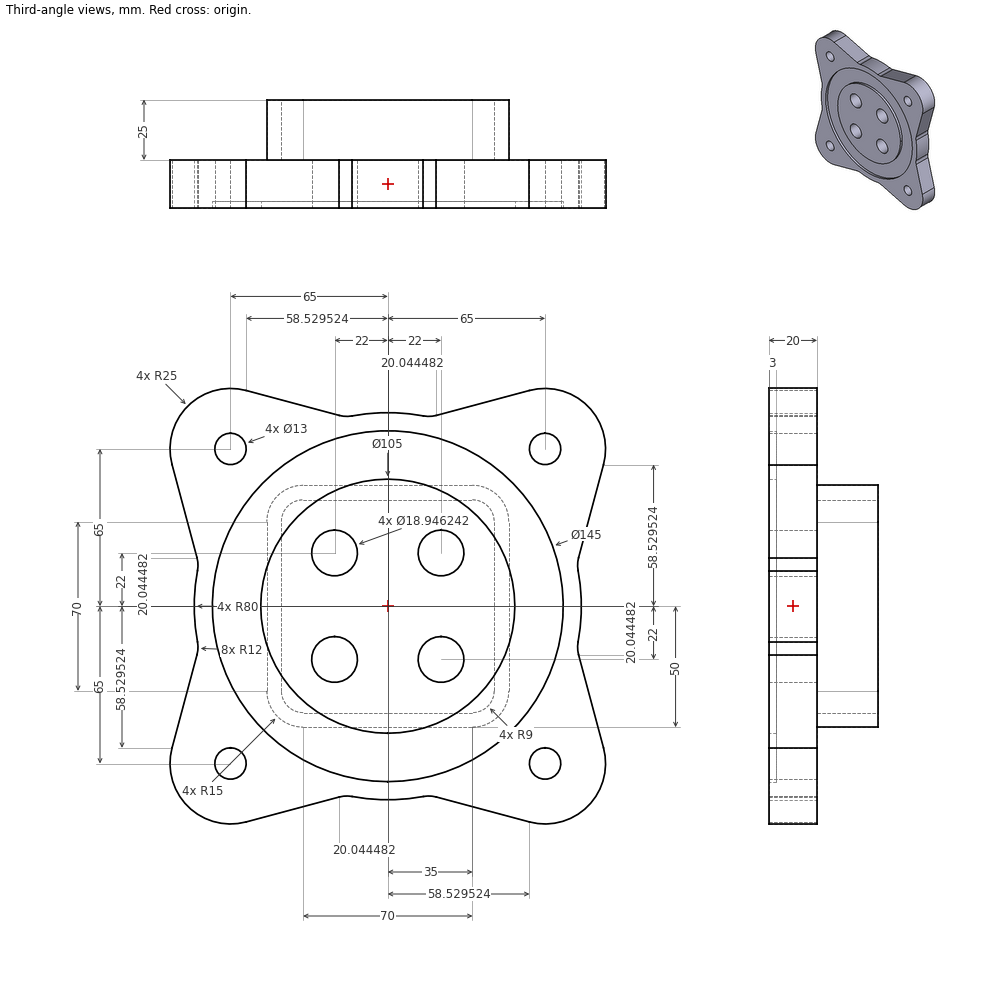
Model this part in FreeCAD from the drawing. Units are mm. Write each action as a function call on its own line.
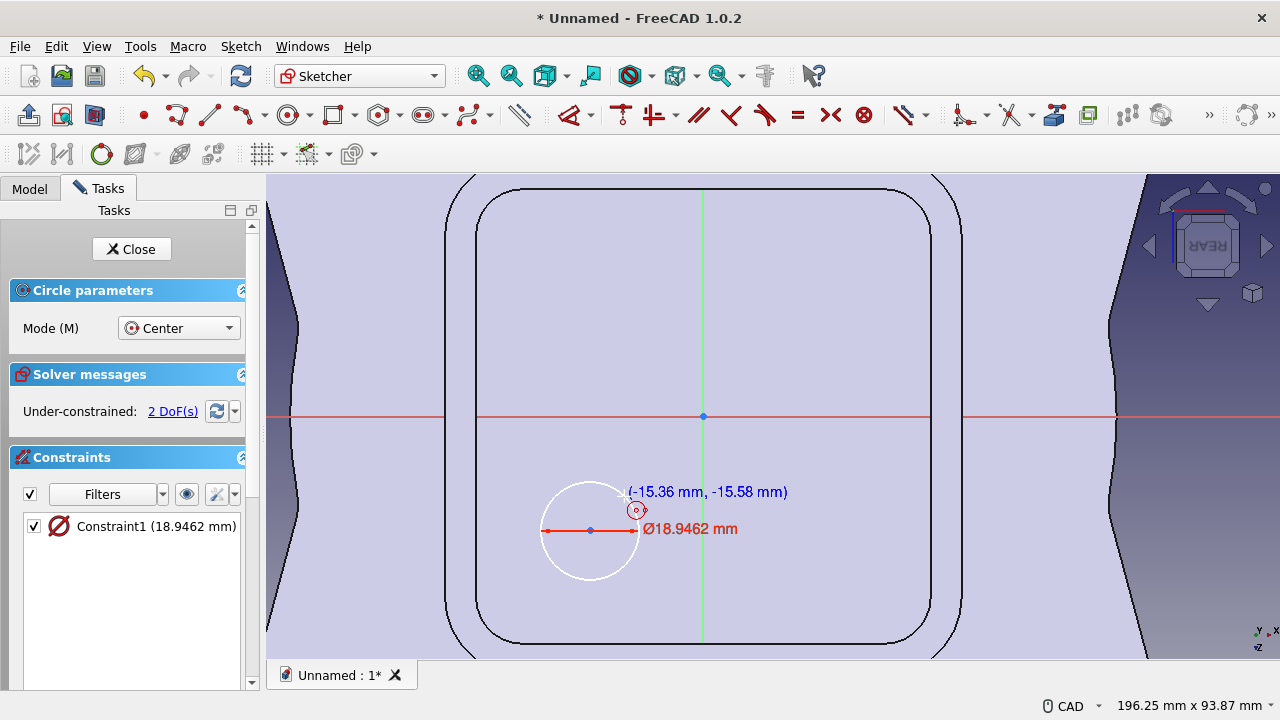
click(817, 530)
move(852, 496)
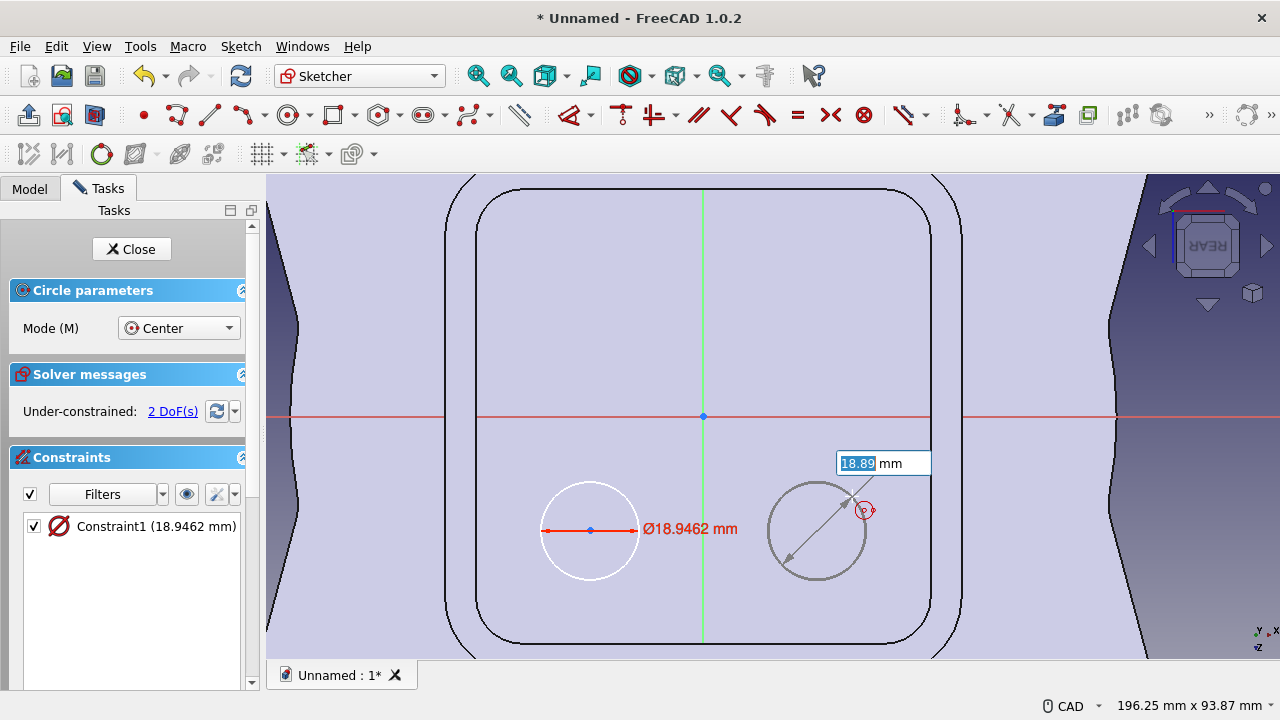
text(18.946242)
key(Return)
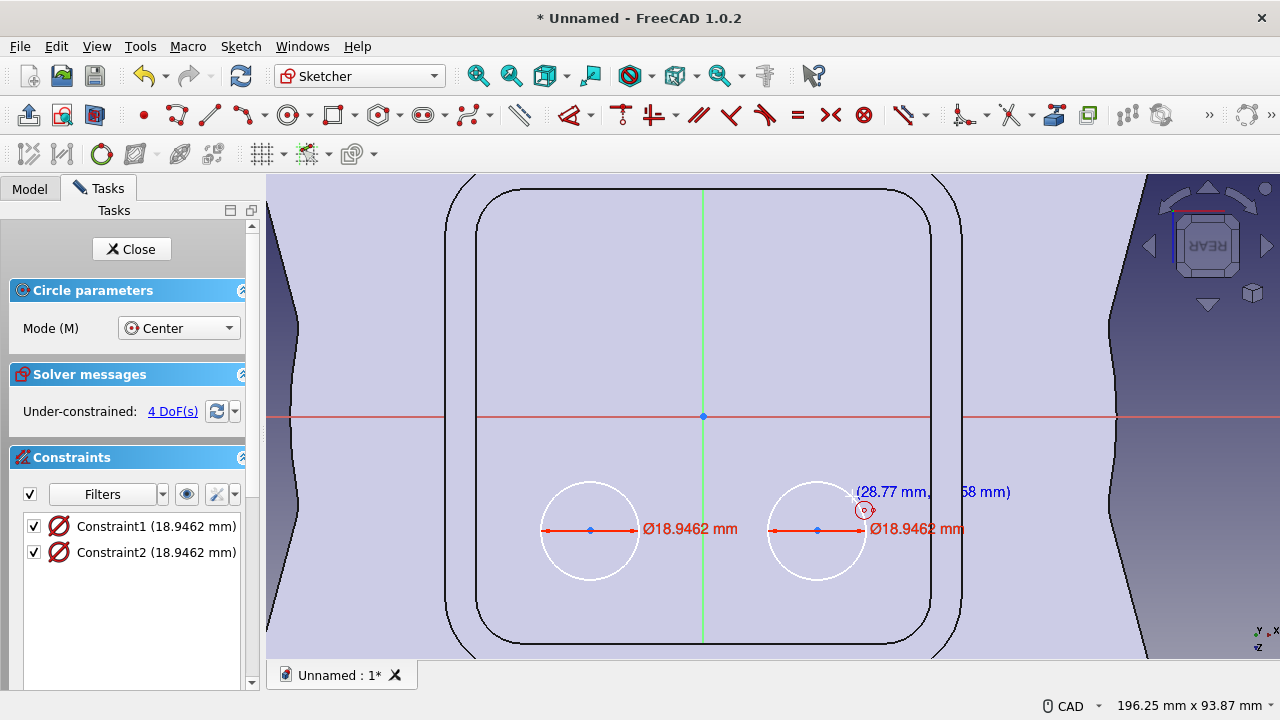
click(817, 303)
move(852, 268)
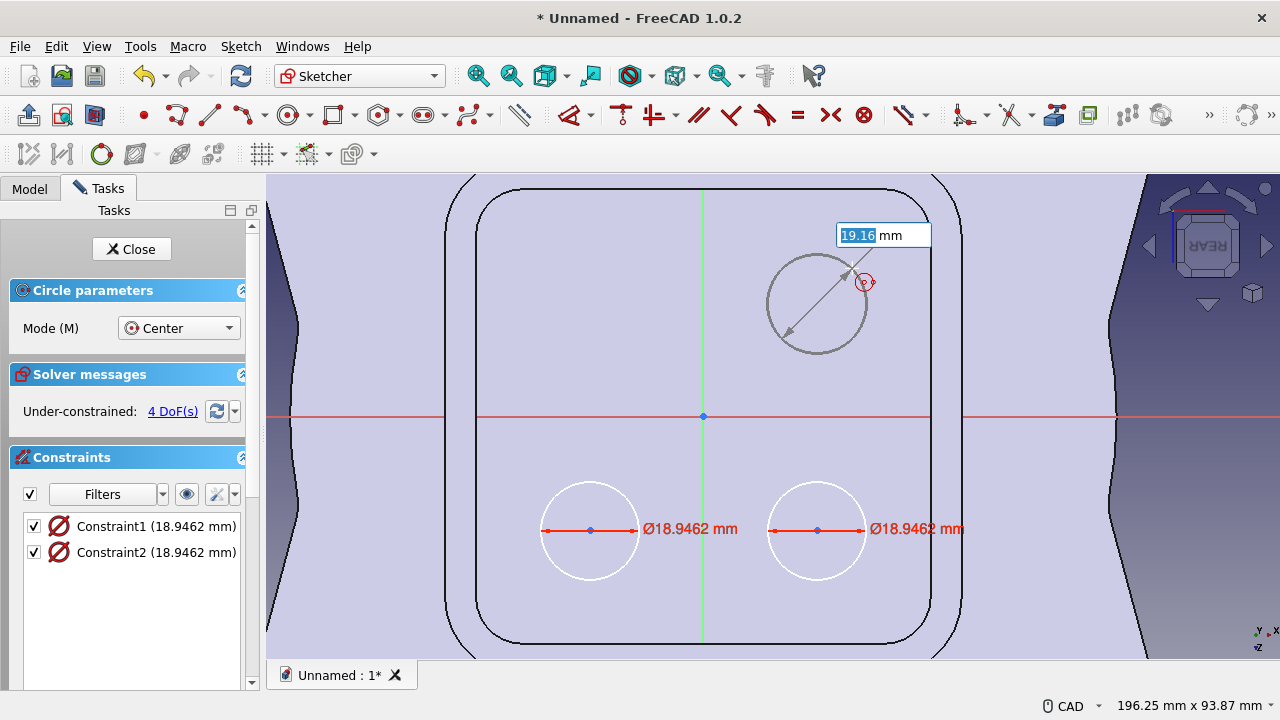
text(18.946242)
key(Return)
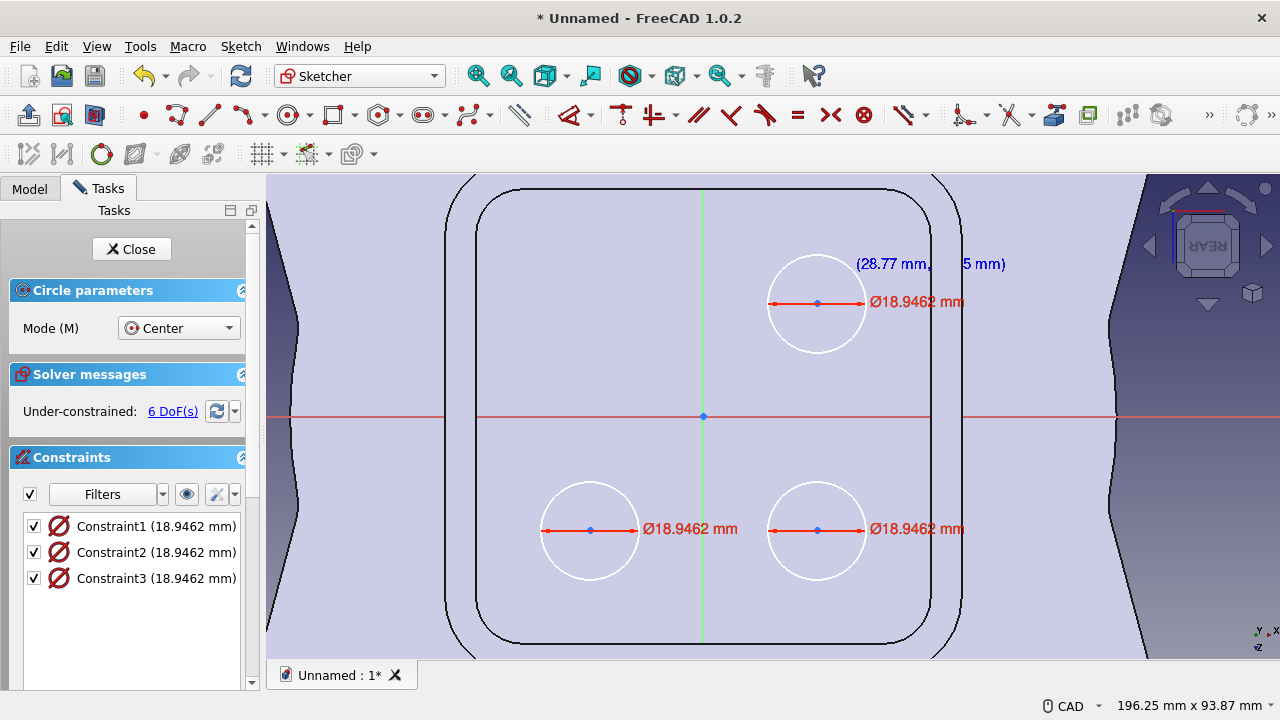
click(590, 303)
move(624, 268)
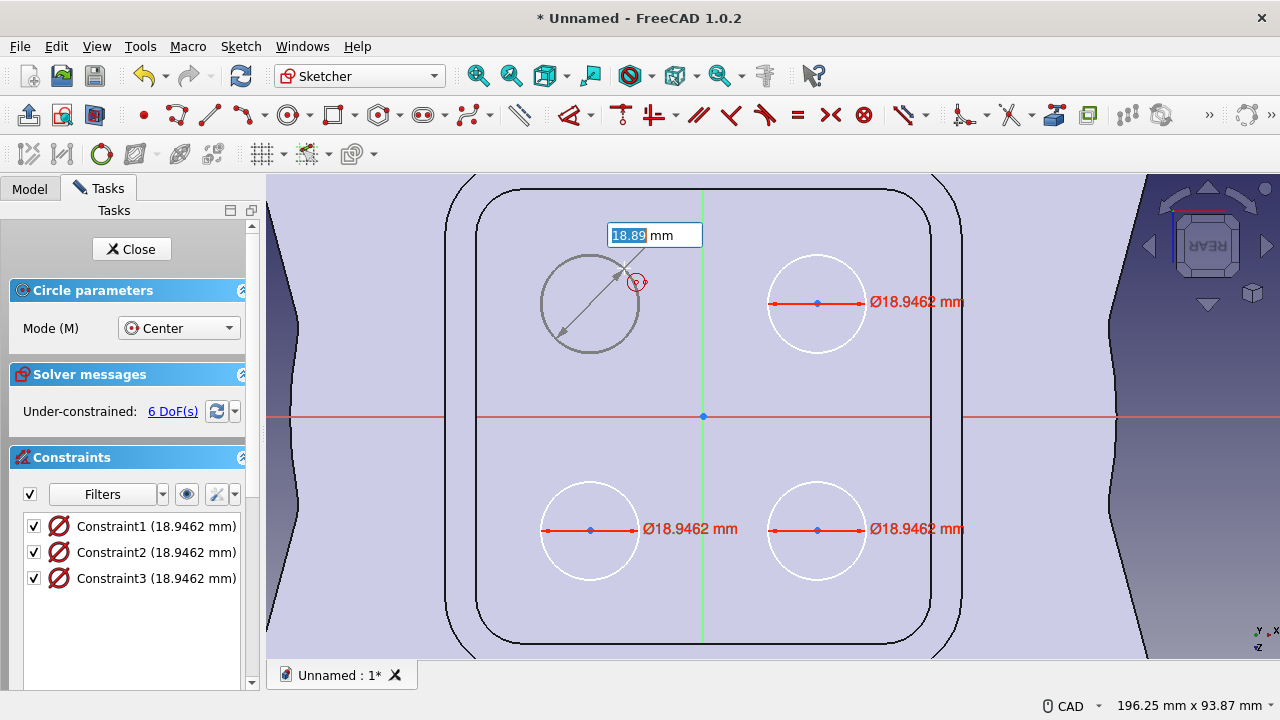
text(18.946242)
key(Return)
key(Escape)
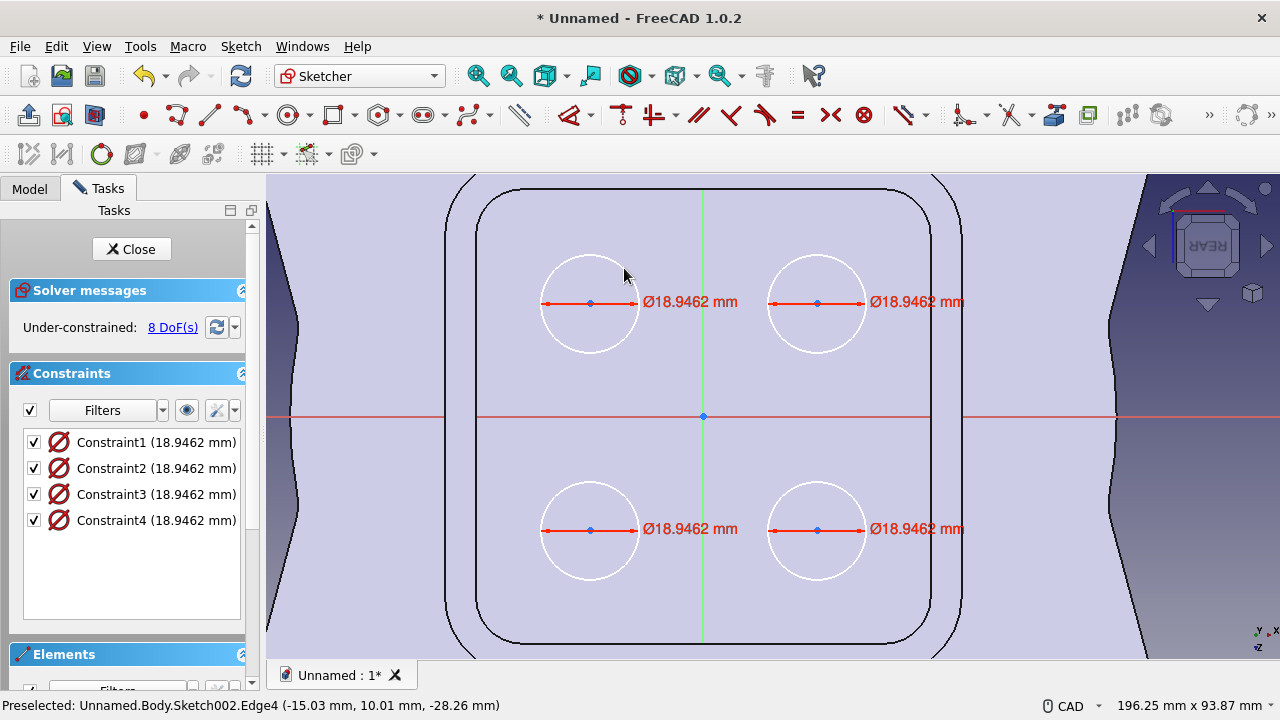
click(590, 531)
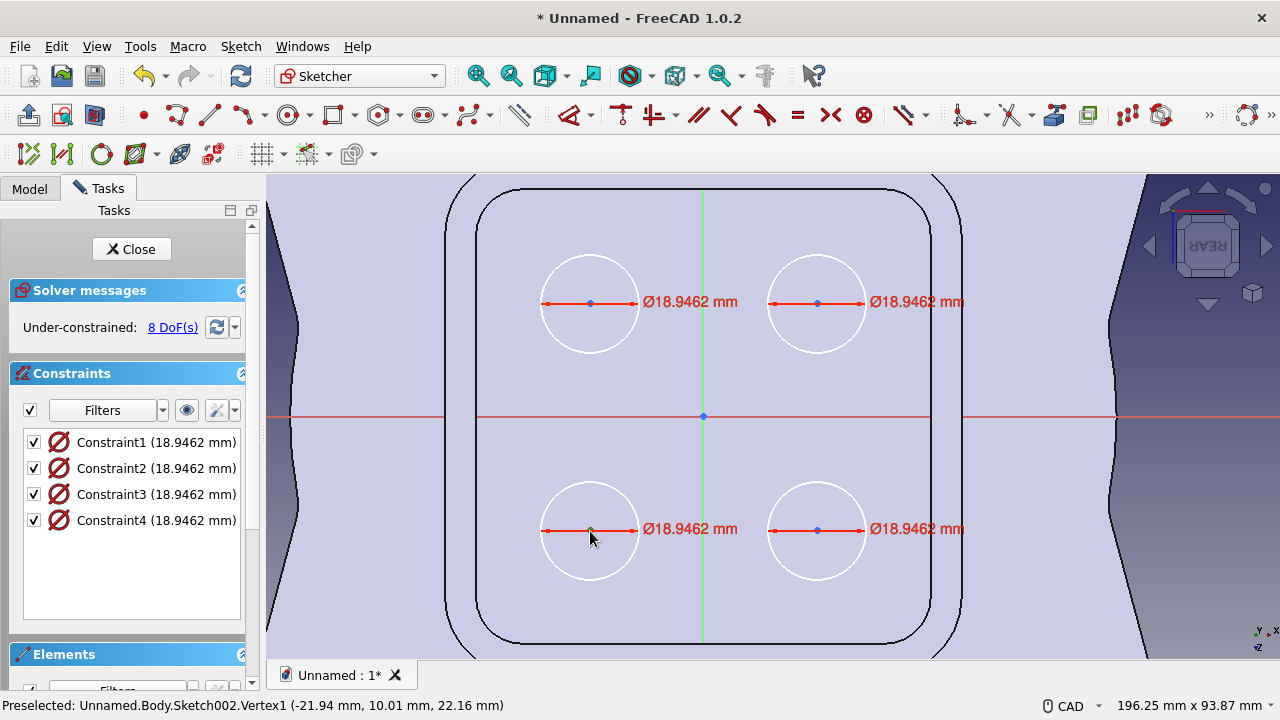
click(817, 531)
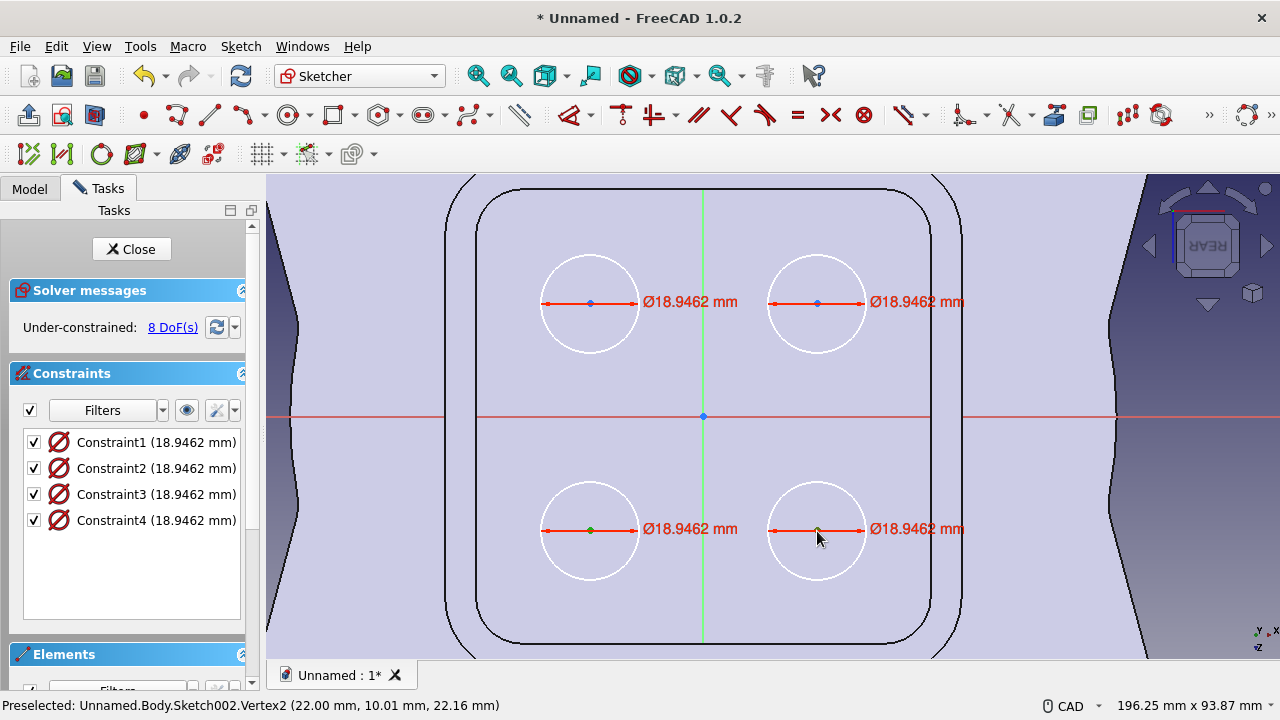
key(h)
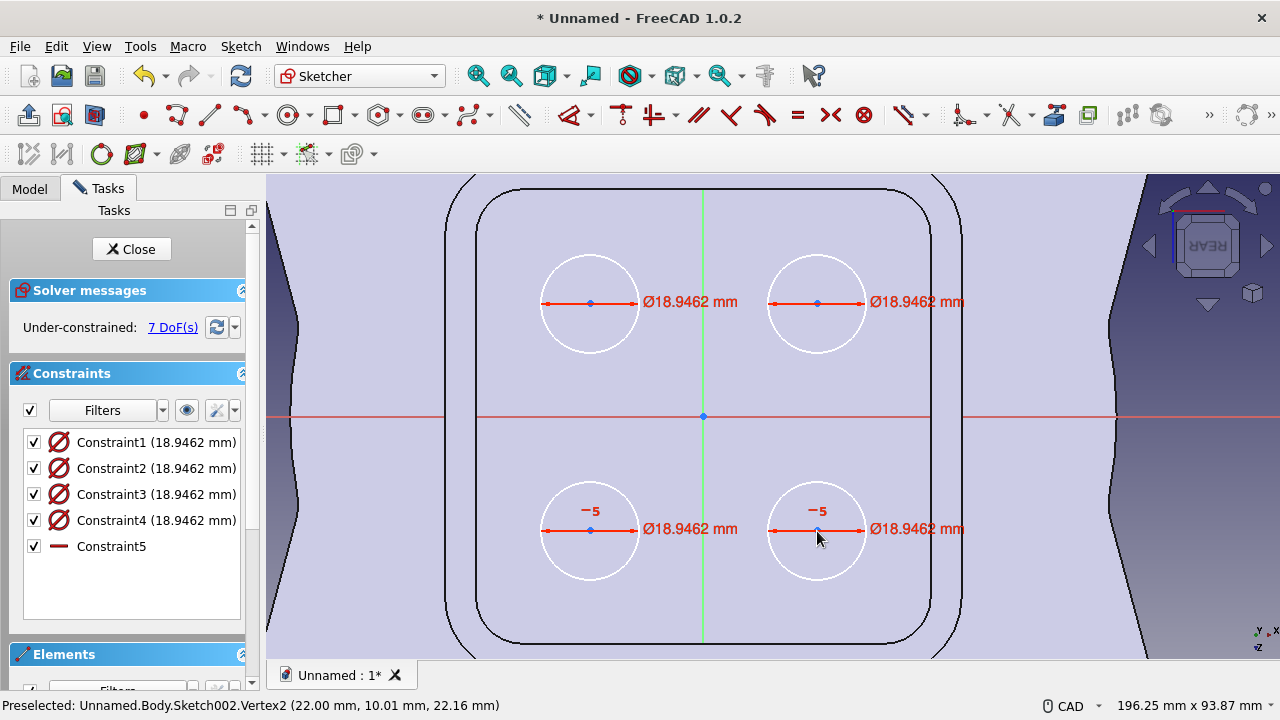
click(817, 531)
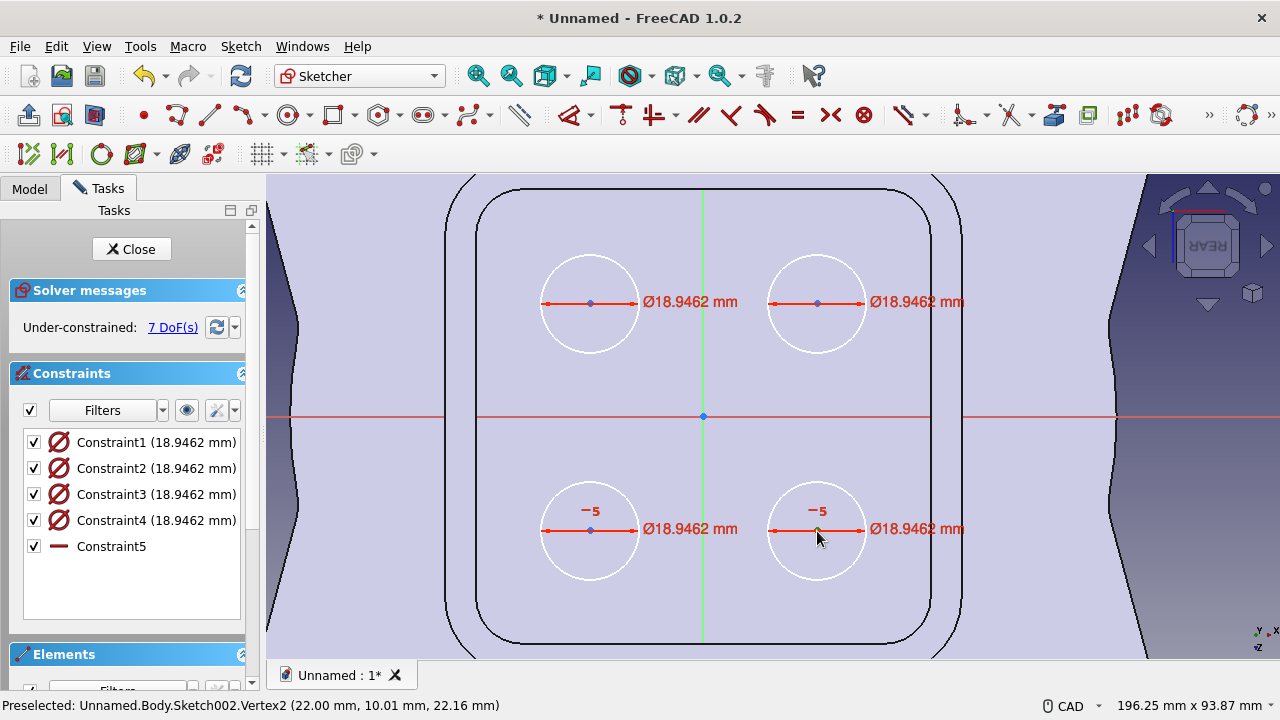
click(817, 304)